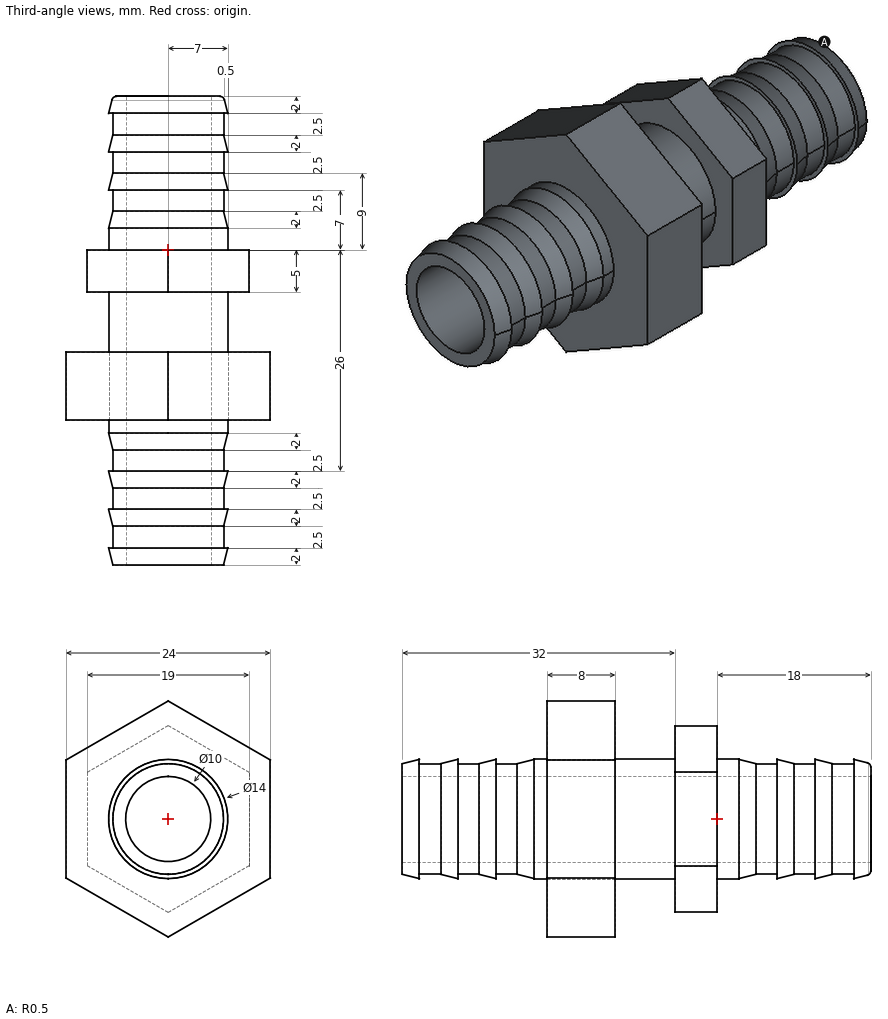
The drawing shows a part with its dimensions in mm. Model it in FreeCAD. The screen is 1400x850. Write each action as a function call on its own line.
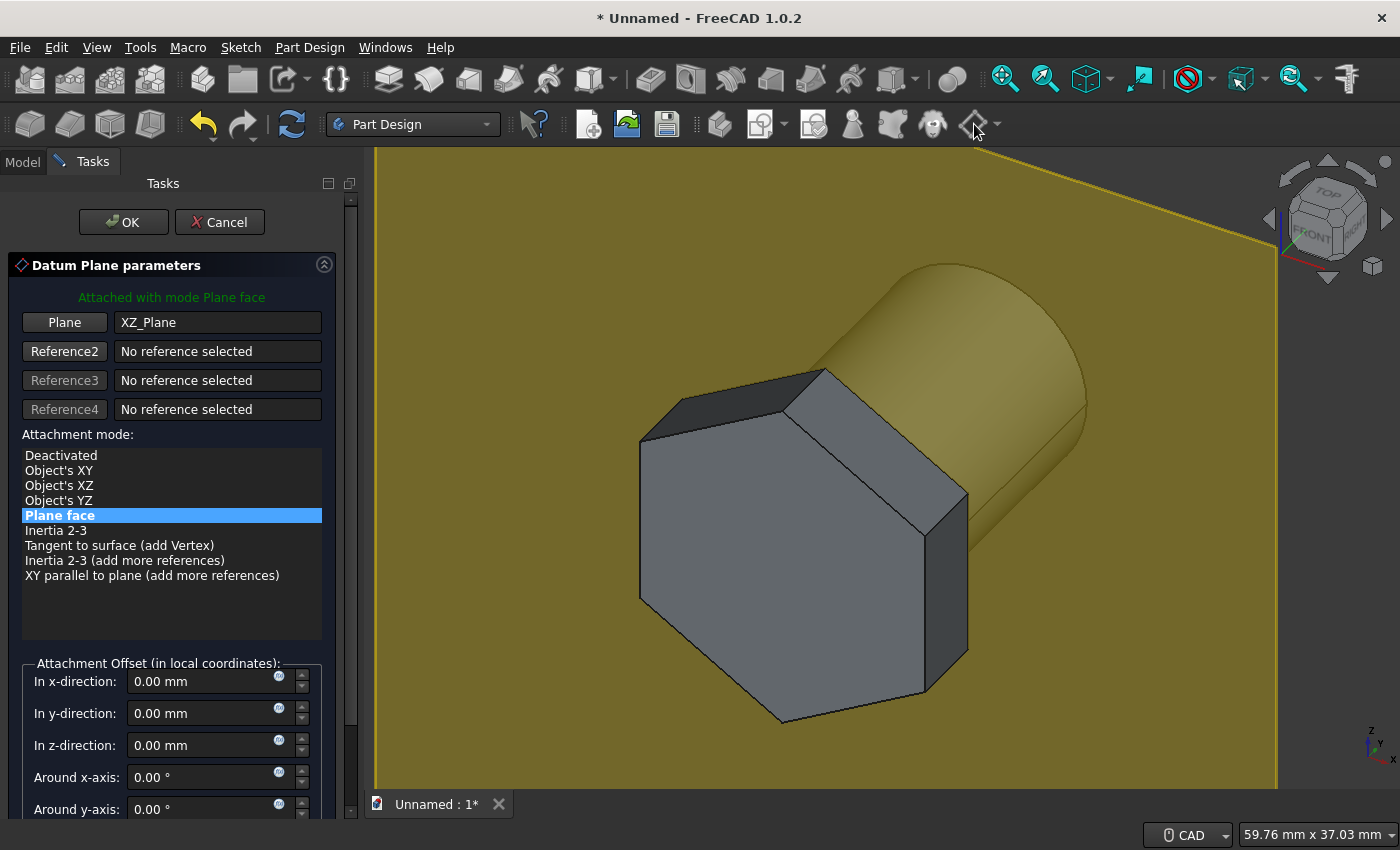
triple_click(210, 745)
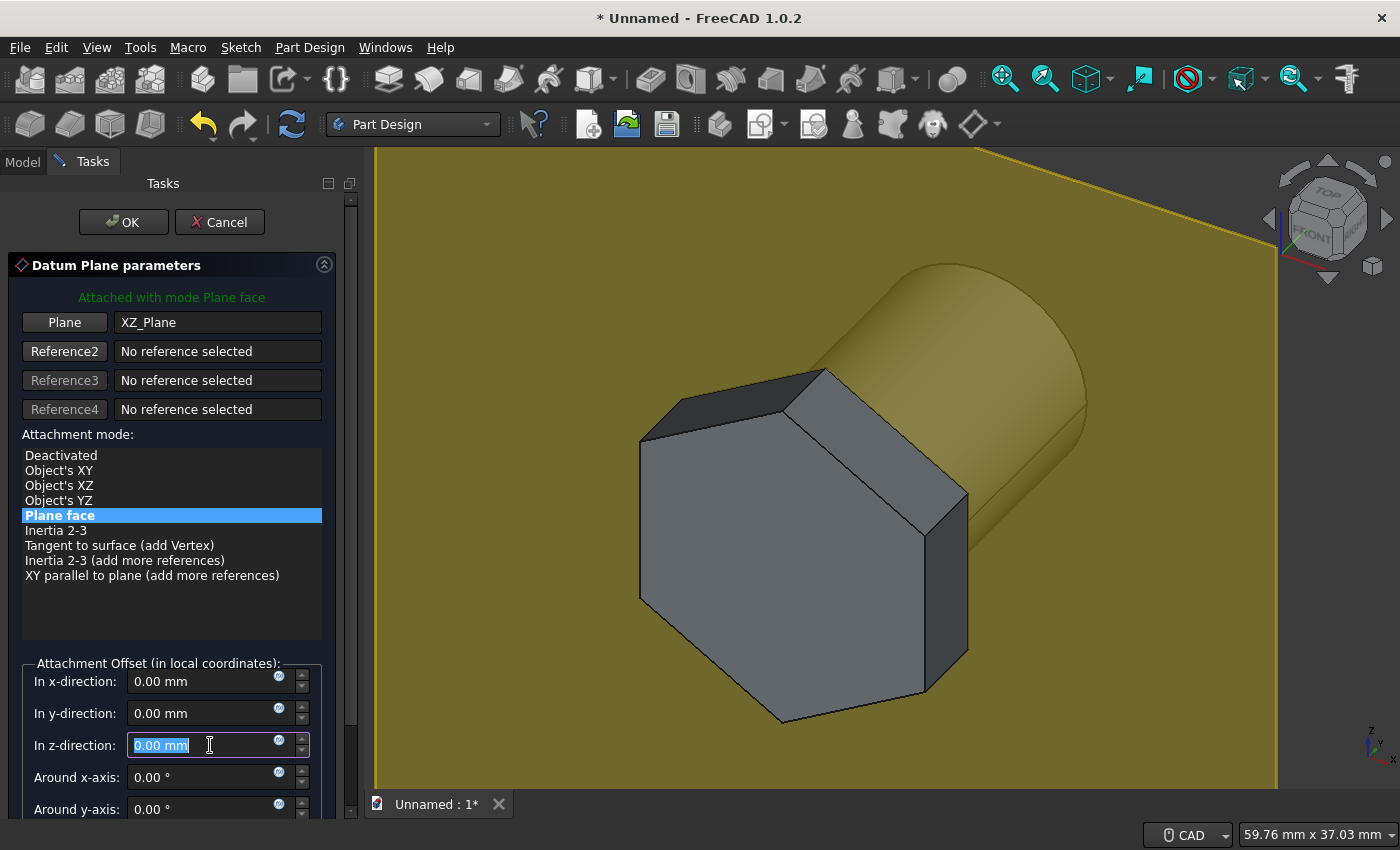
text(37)
key(Tab)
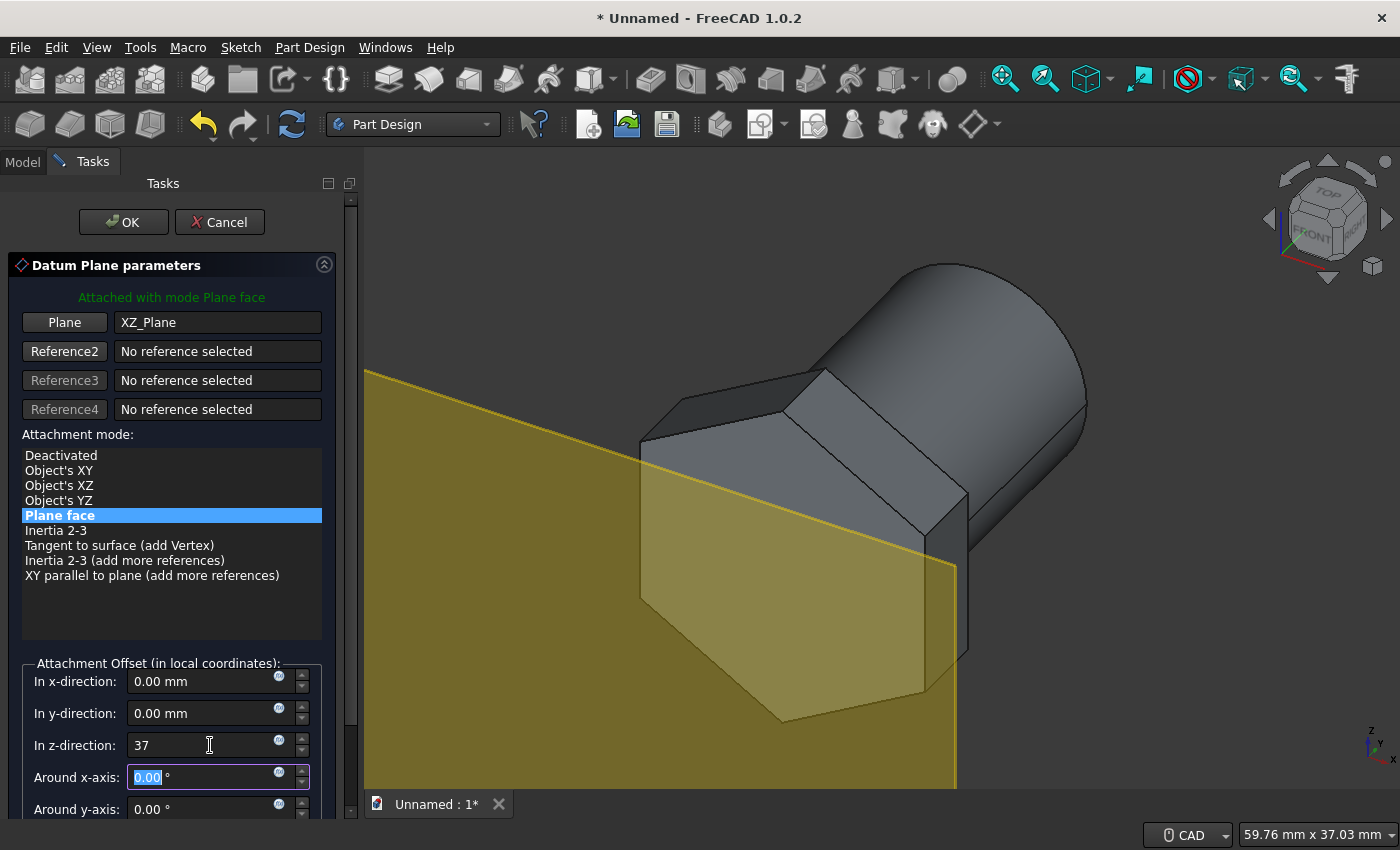
click(124, 222)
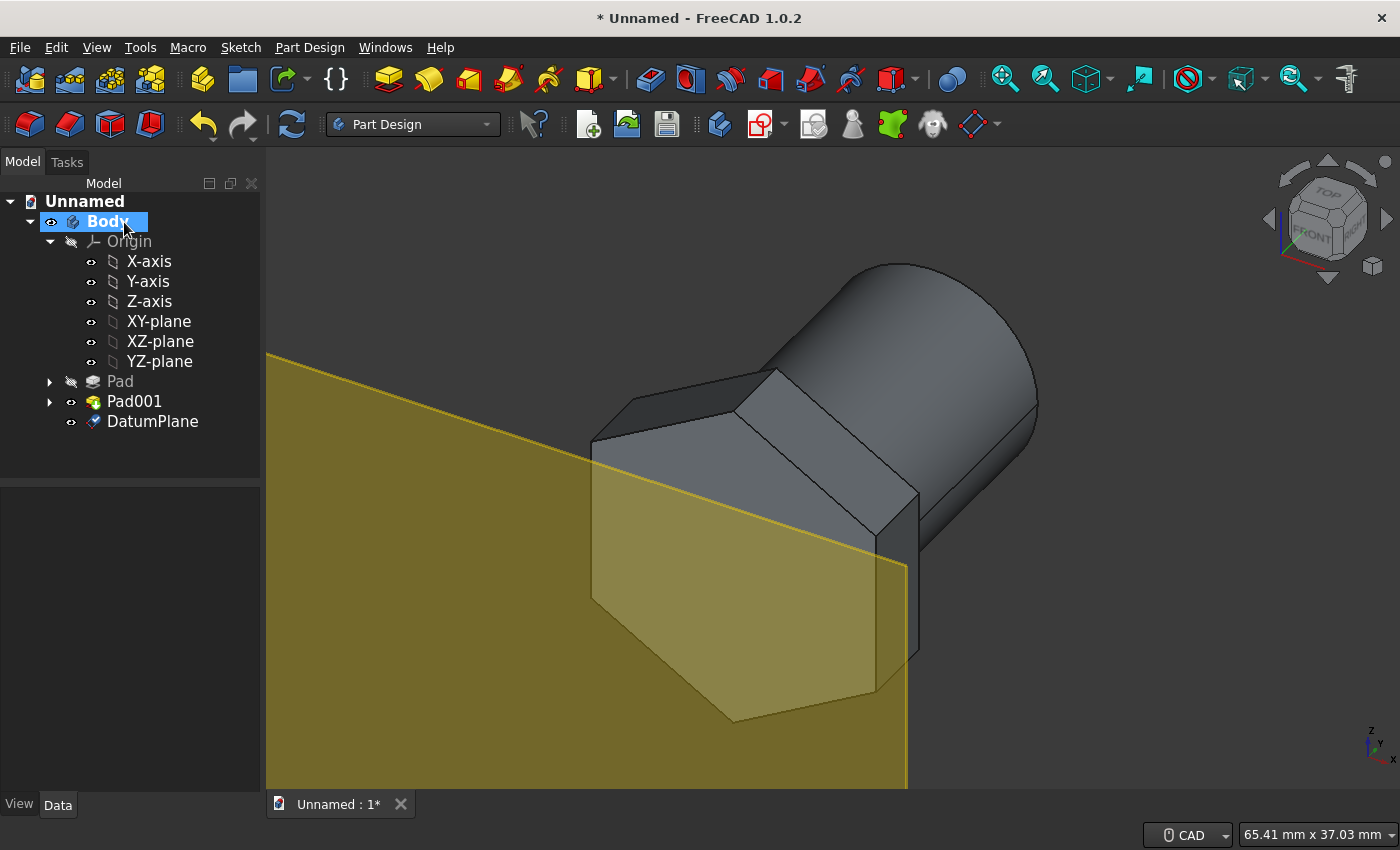
click(116, 422)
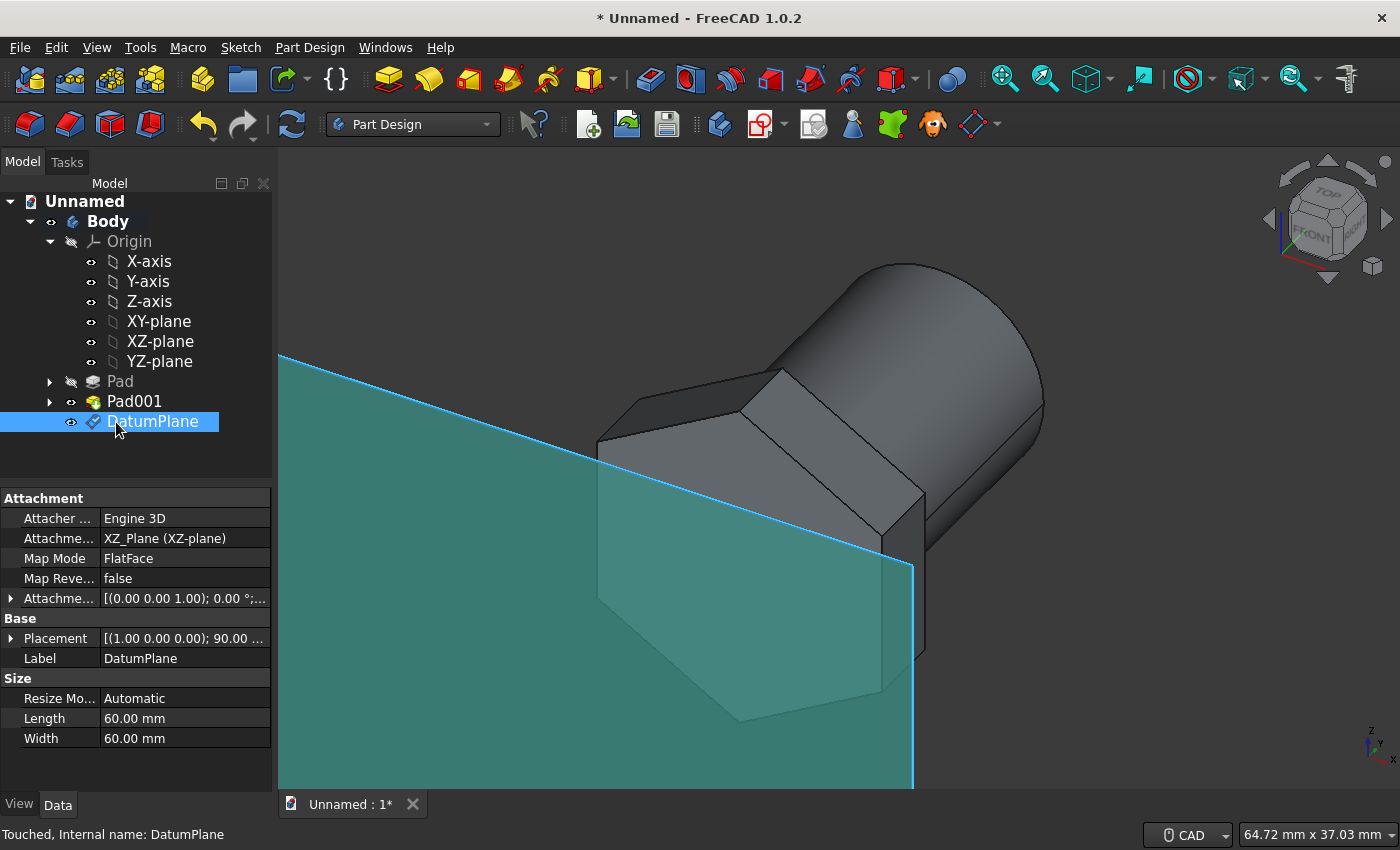
click(760, 124)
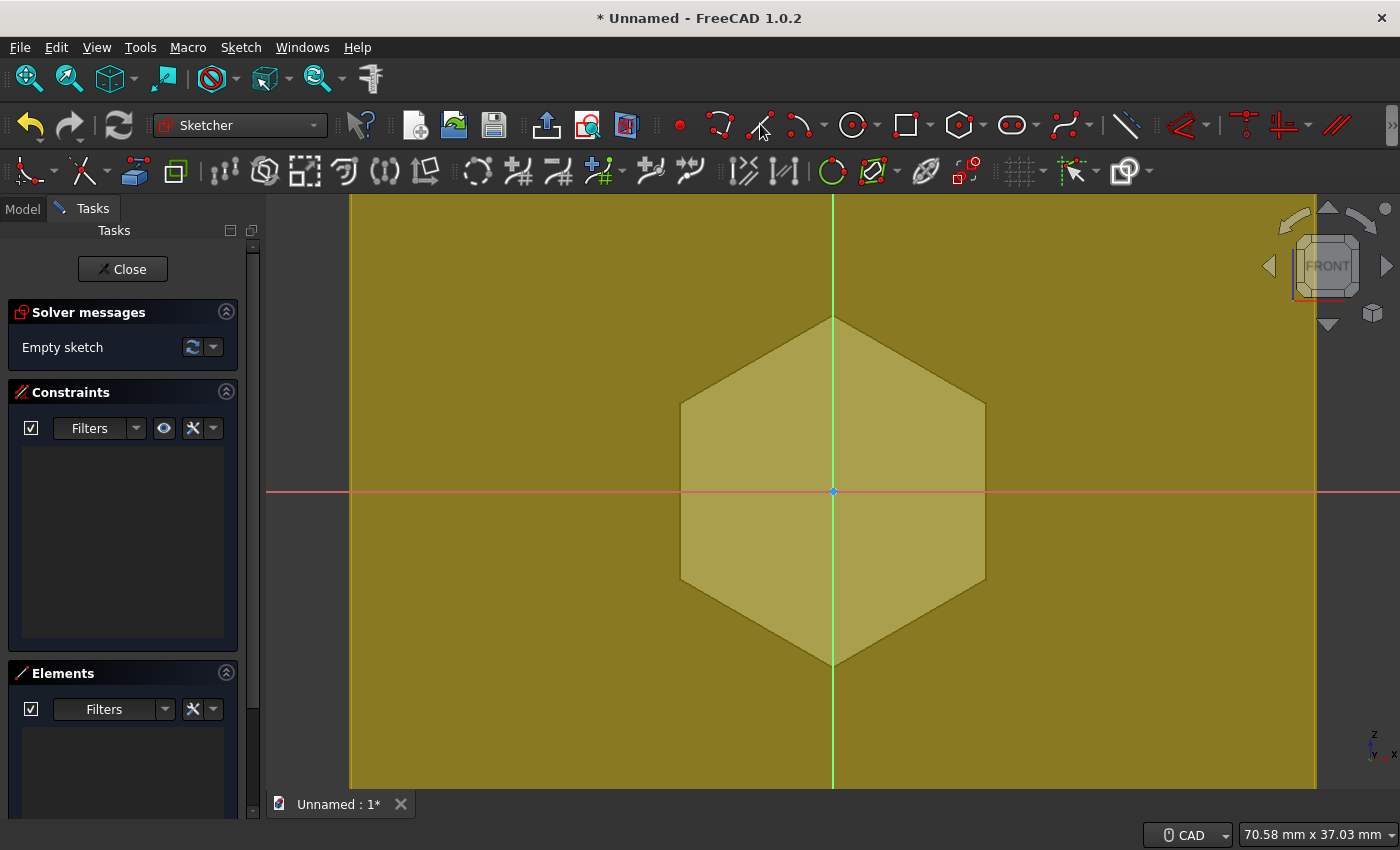
scroll(916, 492, up, 3)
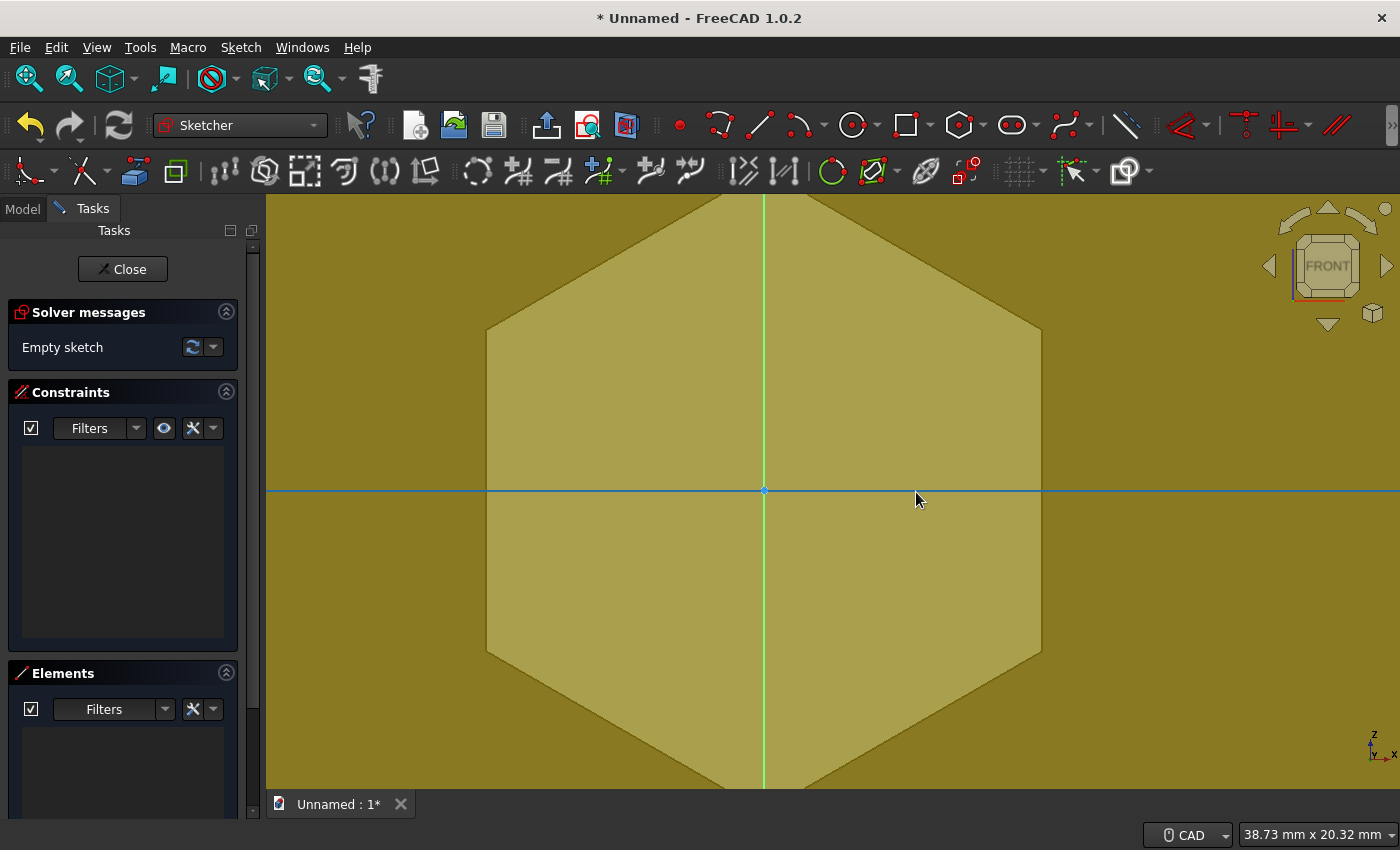
click(854, 126)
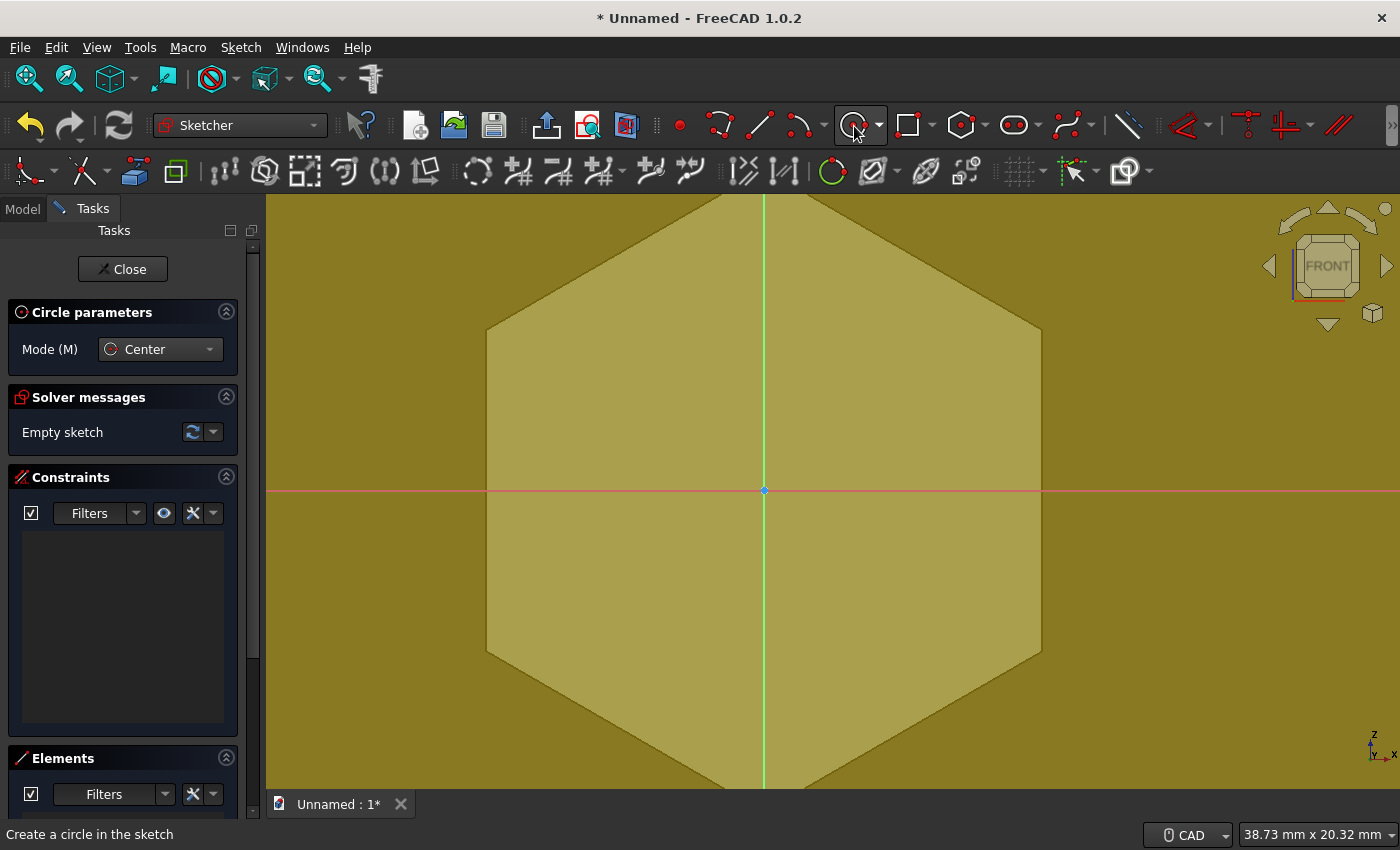
click(764, 491)
move(909, 346)